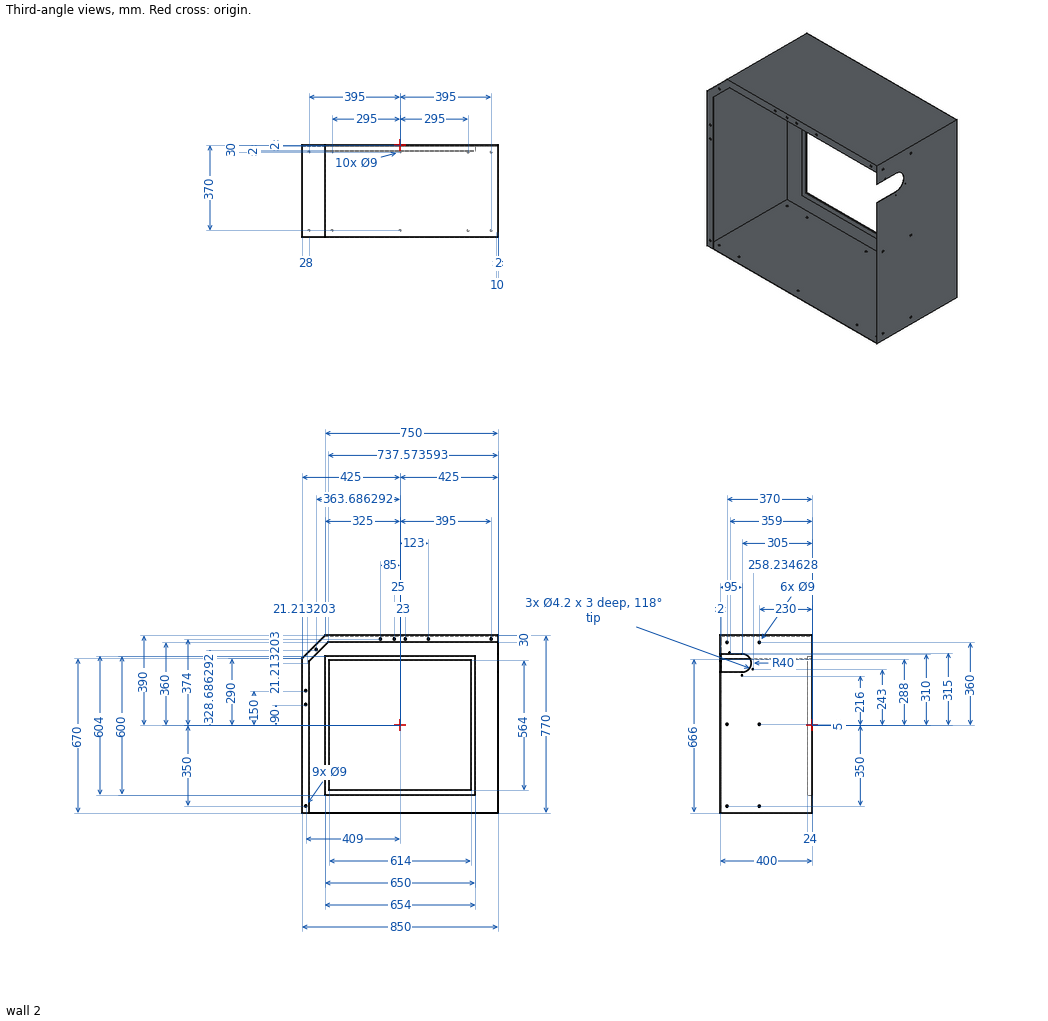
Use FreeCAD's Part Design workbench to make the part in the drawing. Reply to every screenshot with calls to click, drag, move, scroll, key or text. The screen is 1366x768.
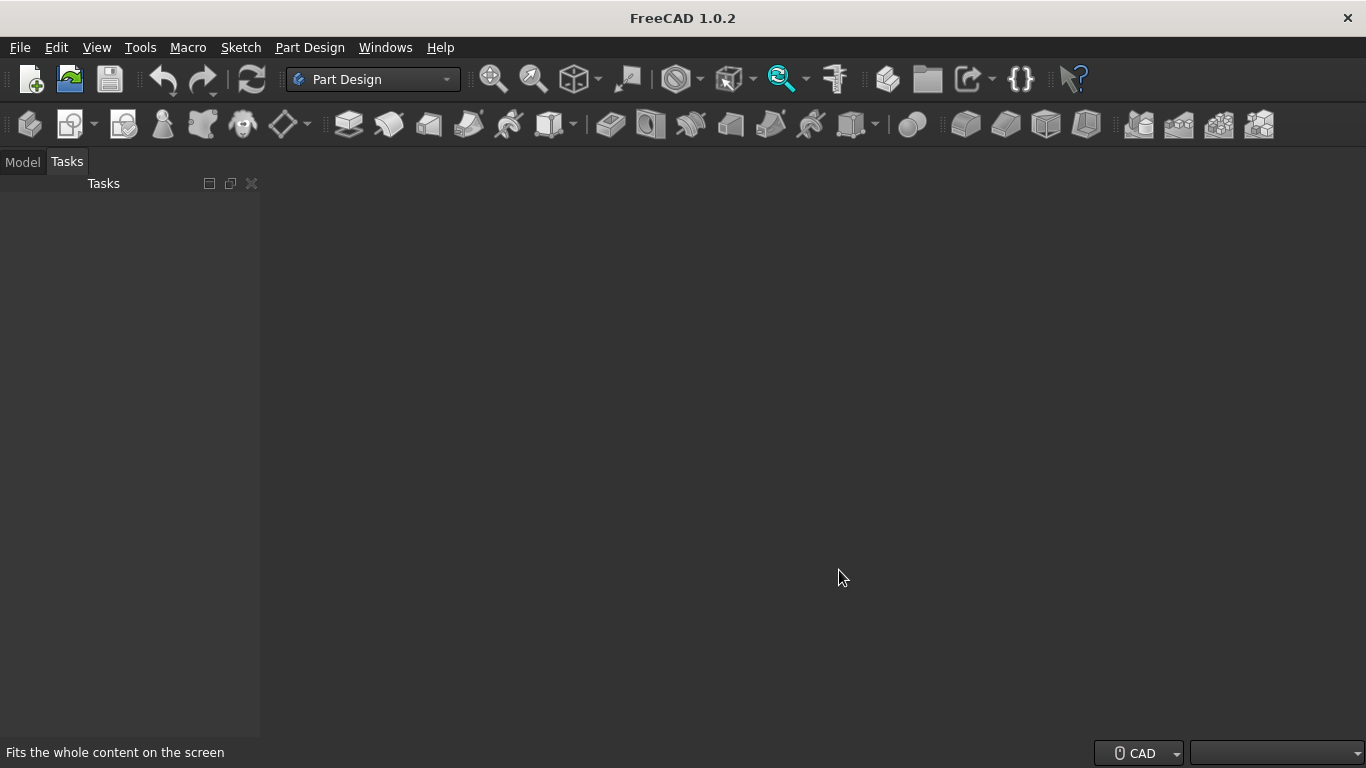
click(30, 80)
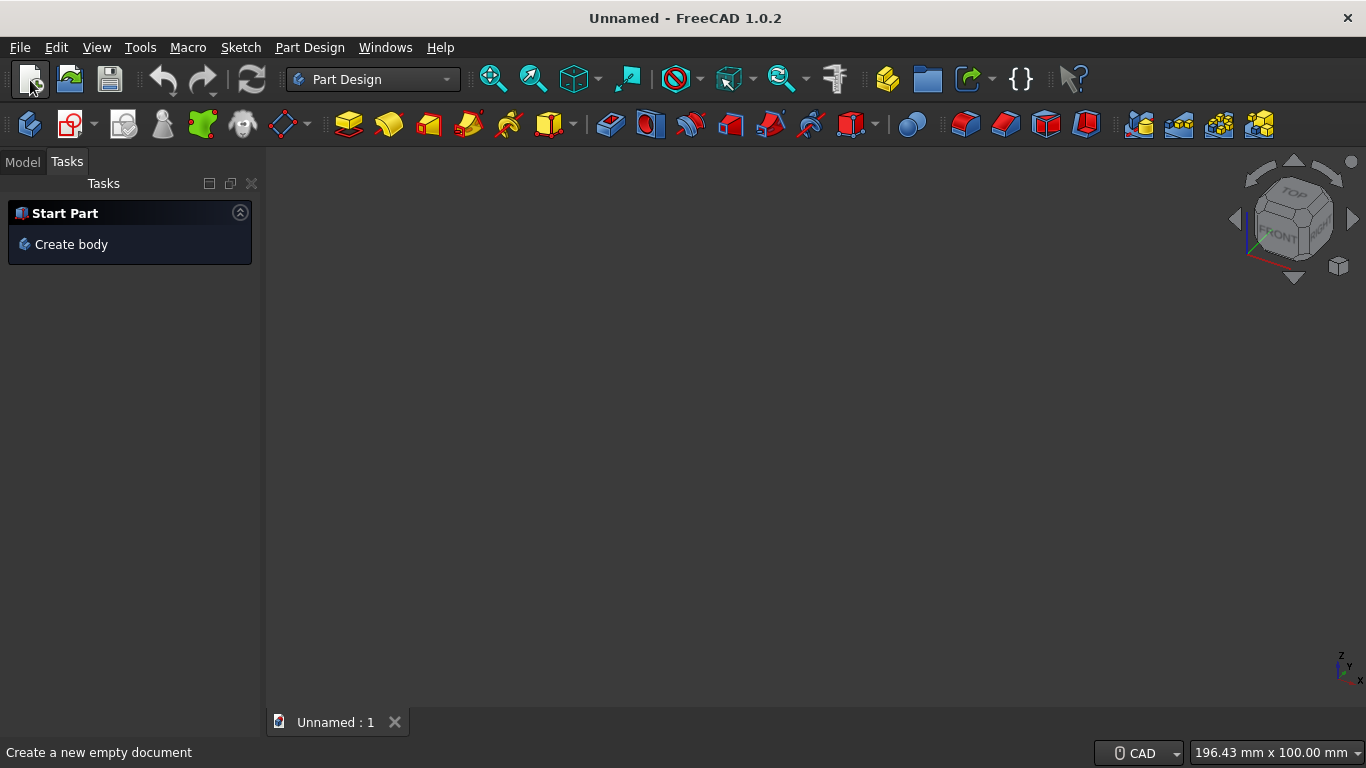
click(70, 124)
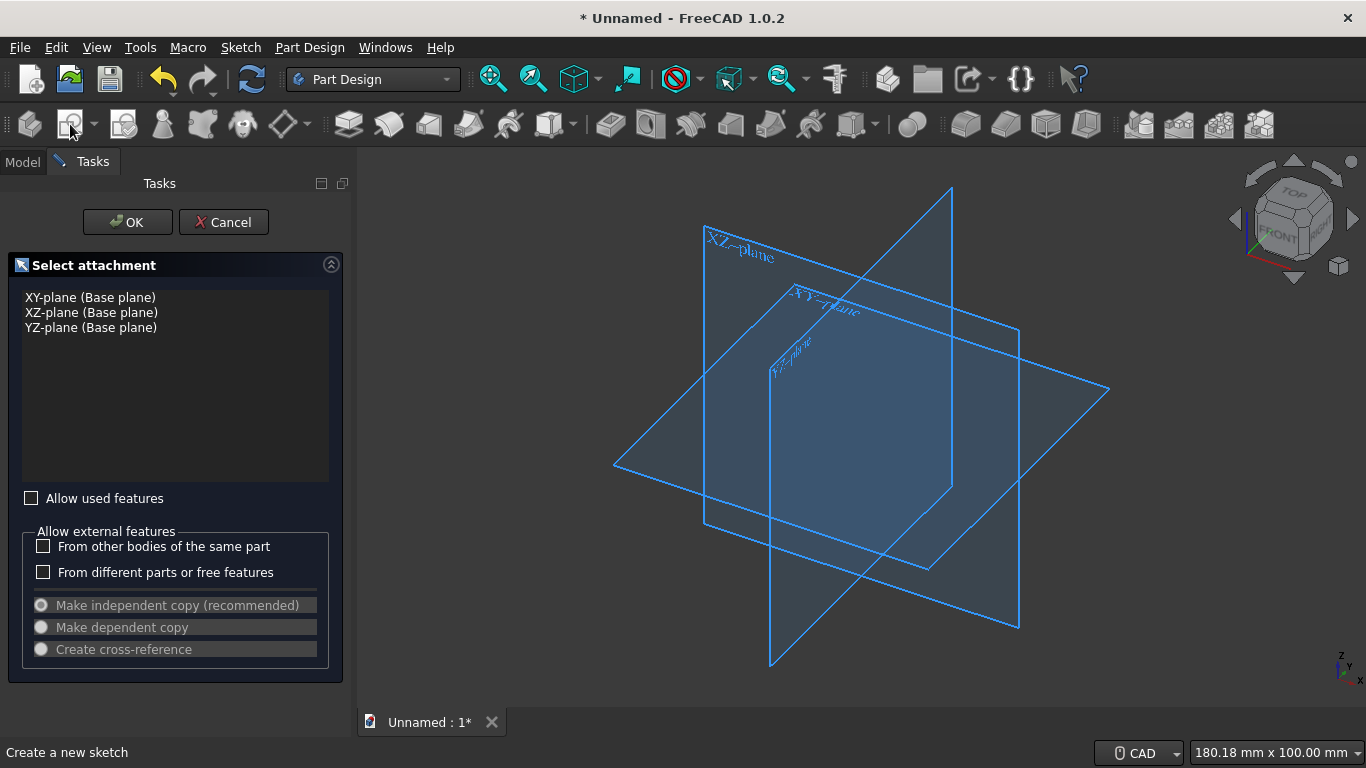
click(82, 312)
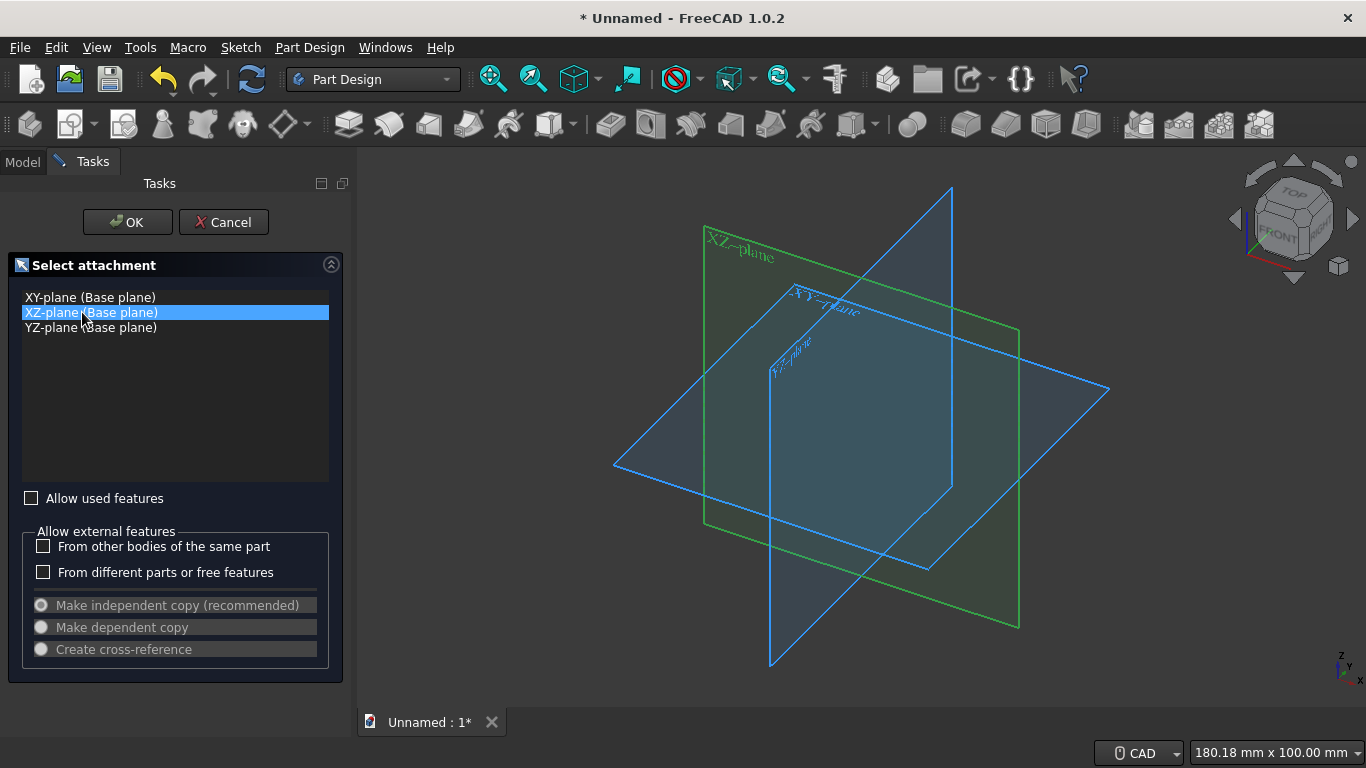
click(128, 222)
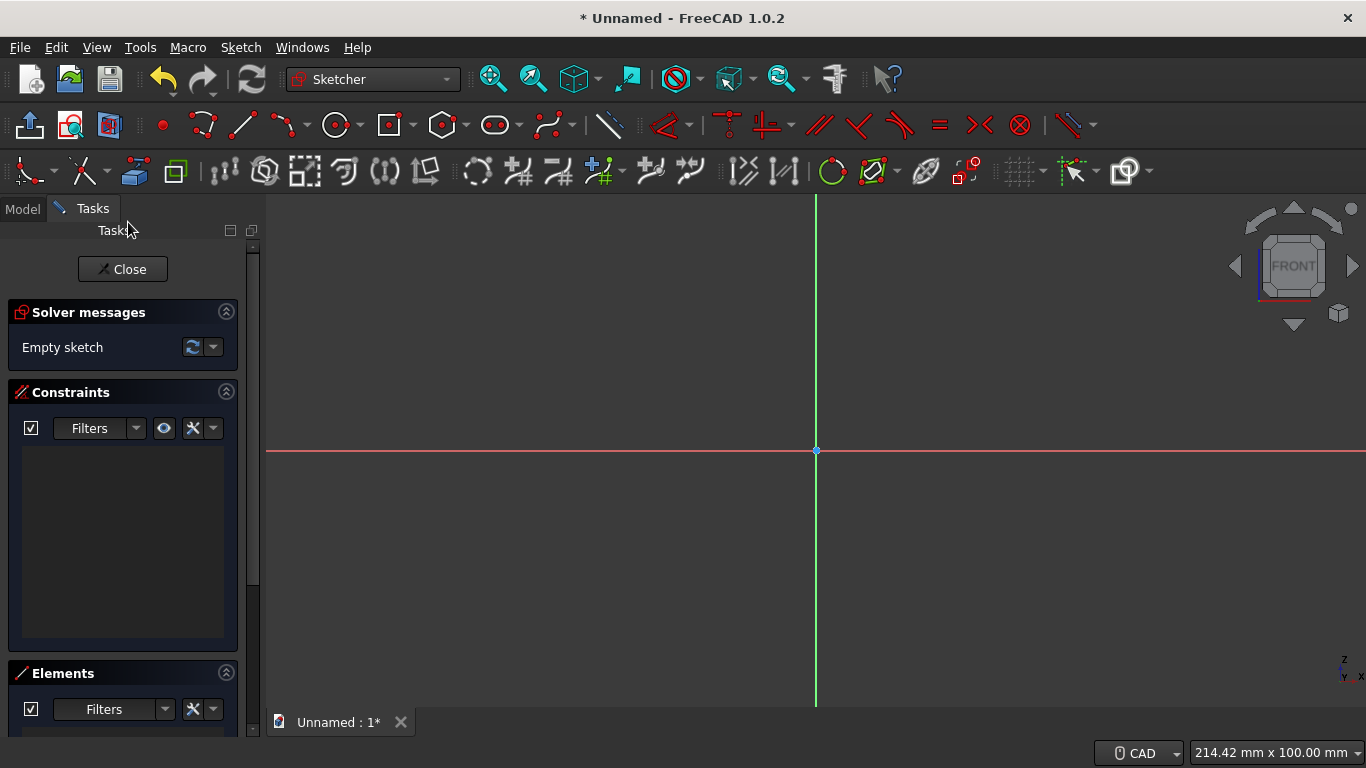
scroll(742, 453, down, 13)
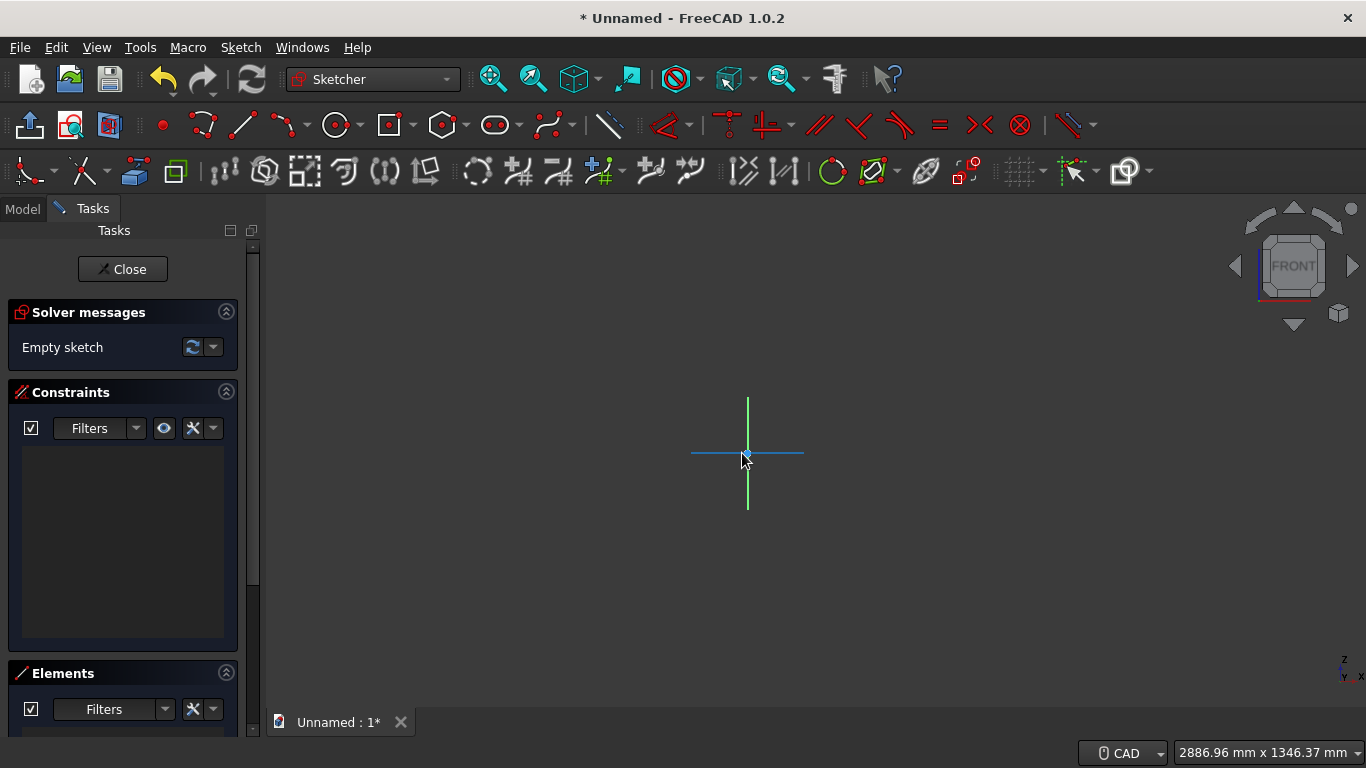
click(204, 126)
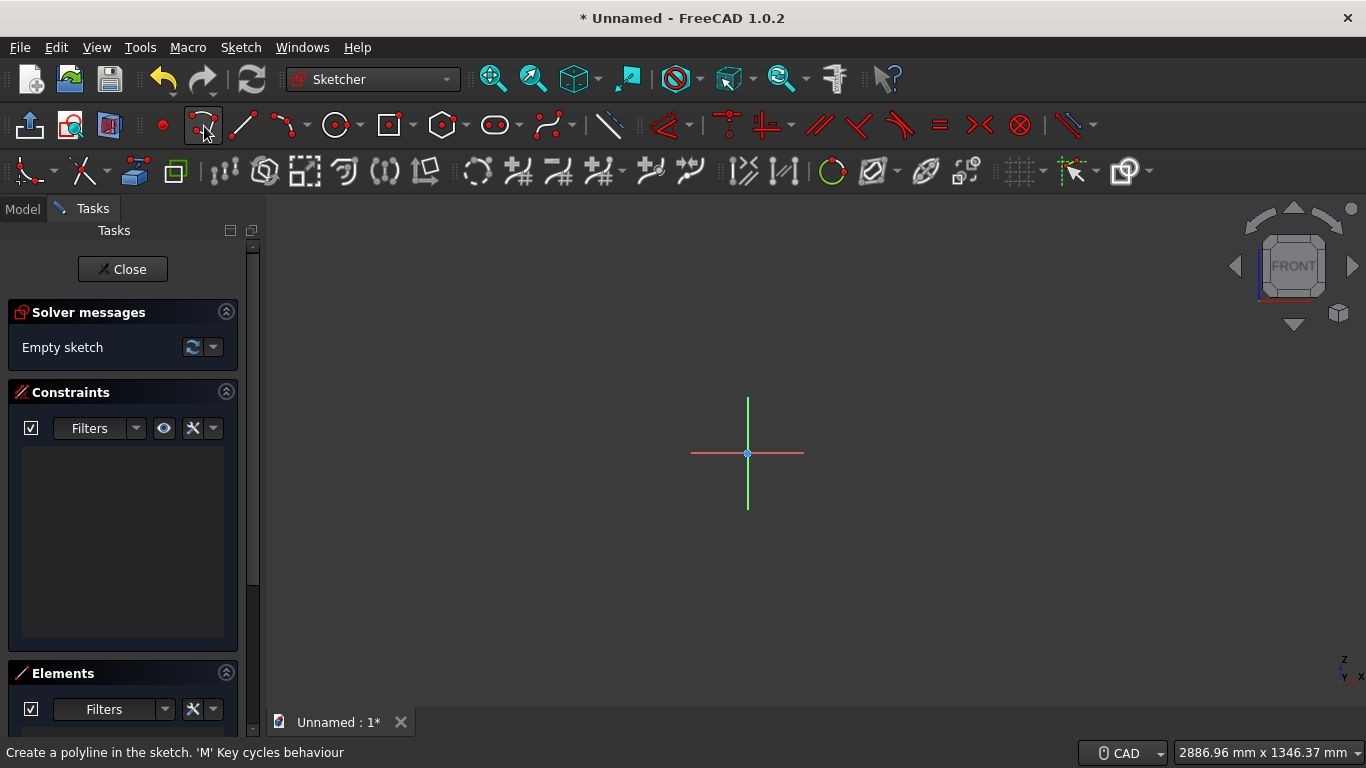
click(624, 305)
click(910, 305)
click(910, 598)
click(586, 598)
click(586, 343)
click(624, 306)
key(Escape)
key(Escape)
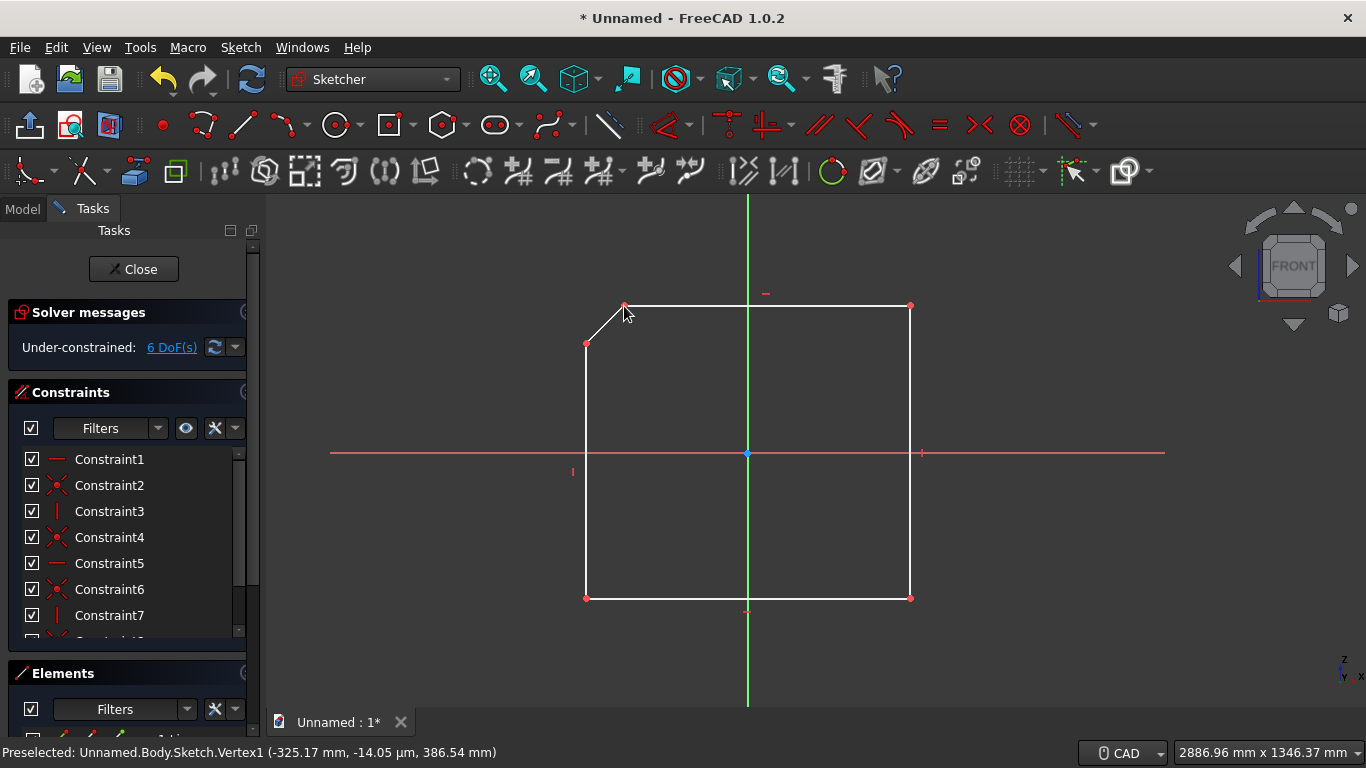
click(664, 126)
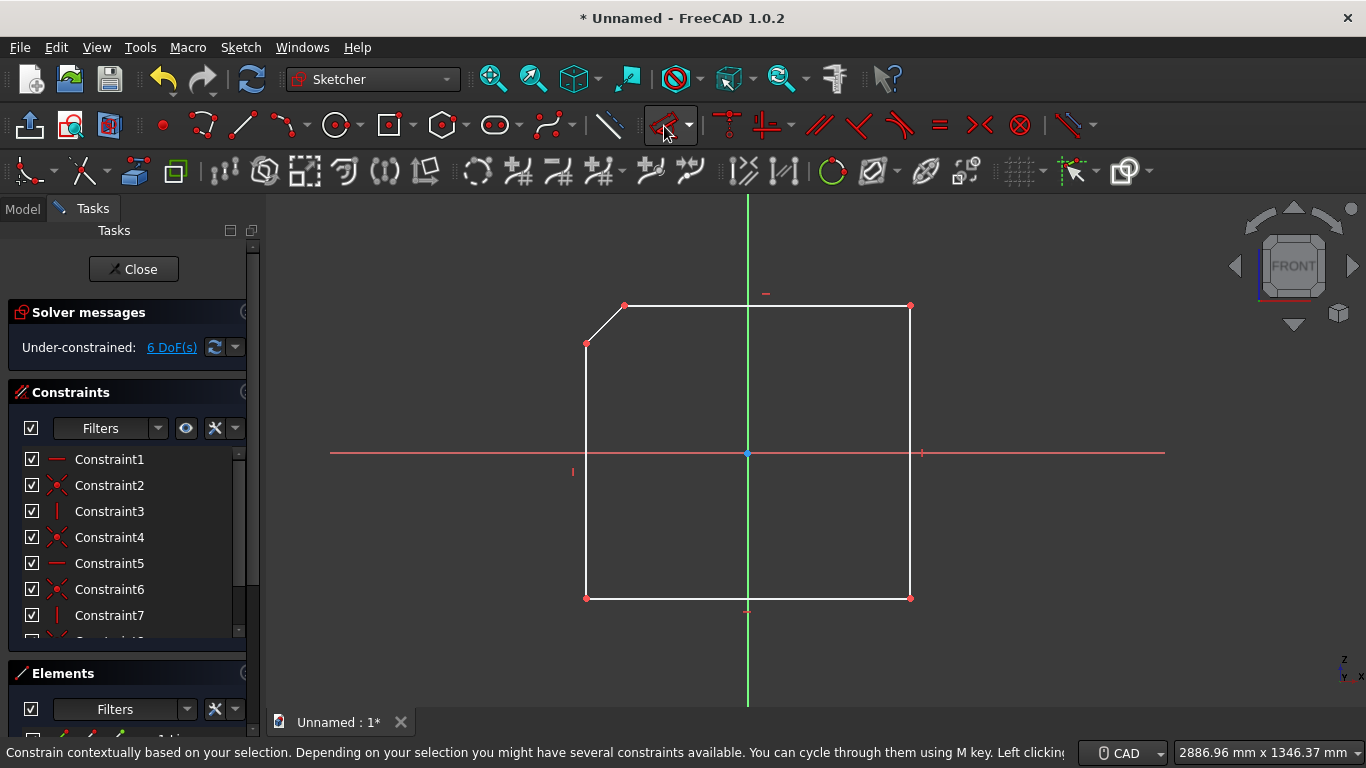
click(710, 306)
click(767, 272)